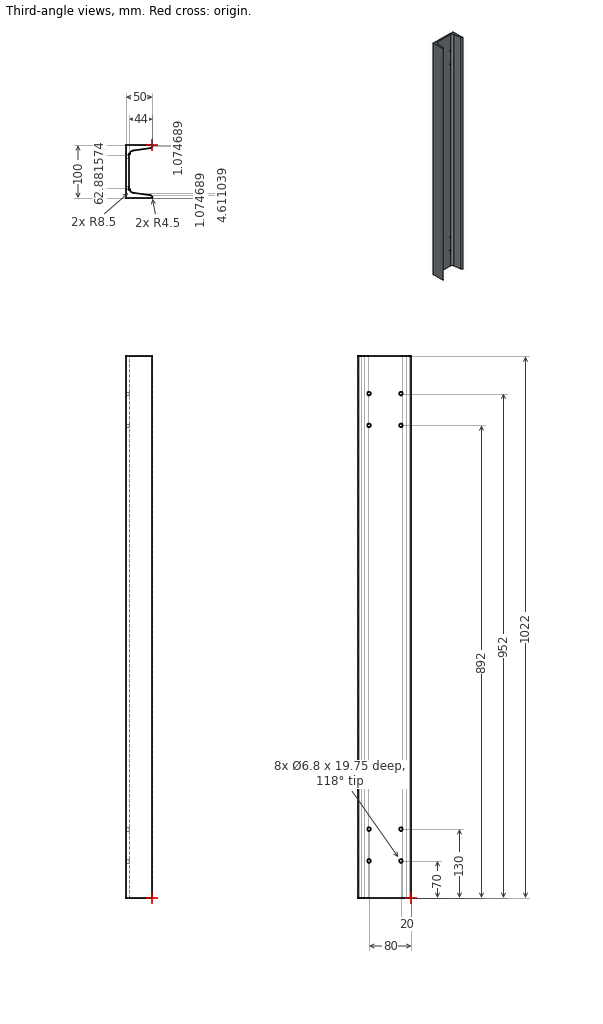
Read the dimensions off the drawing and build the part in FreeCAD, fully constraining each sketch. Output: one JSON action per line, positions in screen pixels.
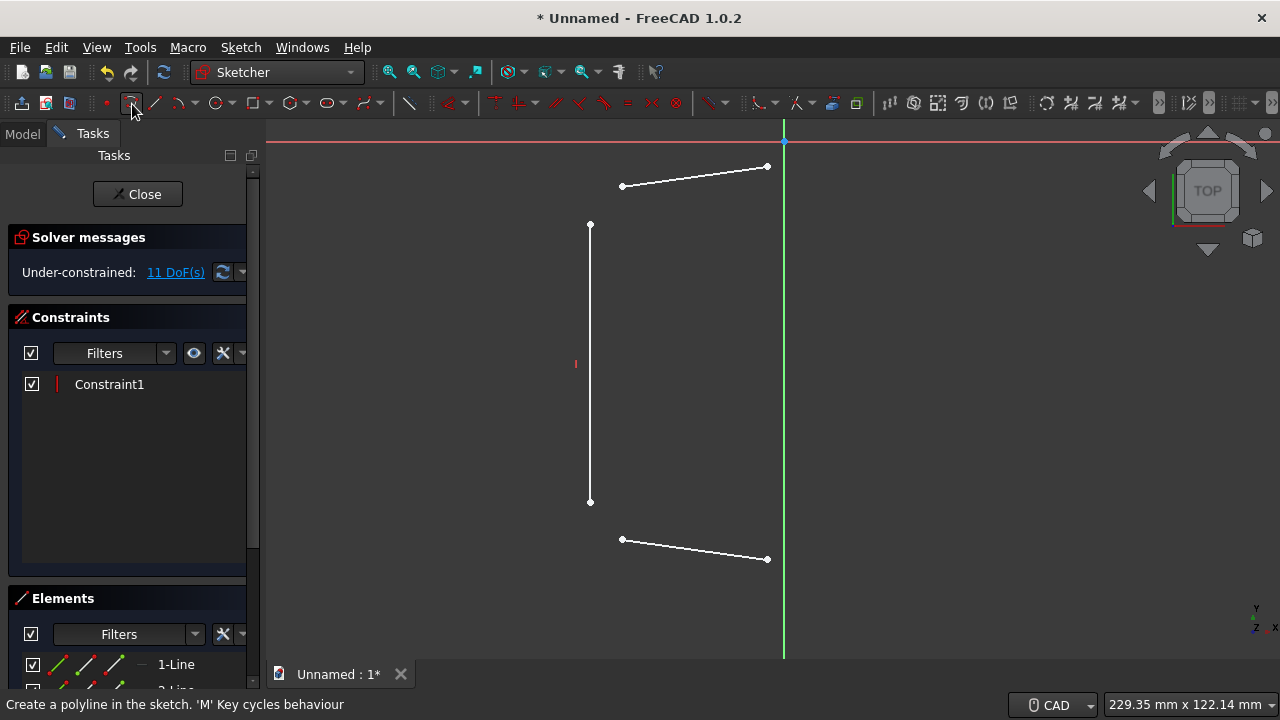
{"action": "scroll", "coordinate": [844, 508], "scroll_direction": "down", "scroll_amount": 1}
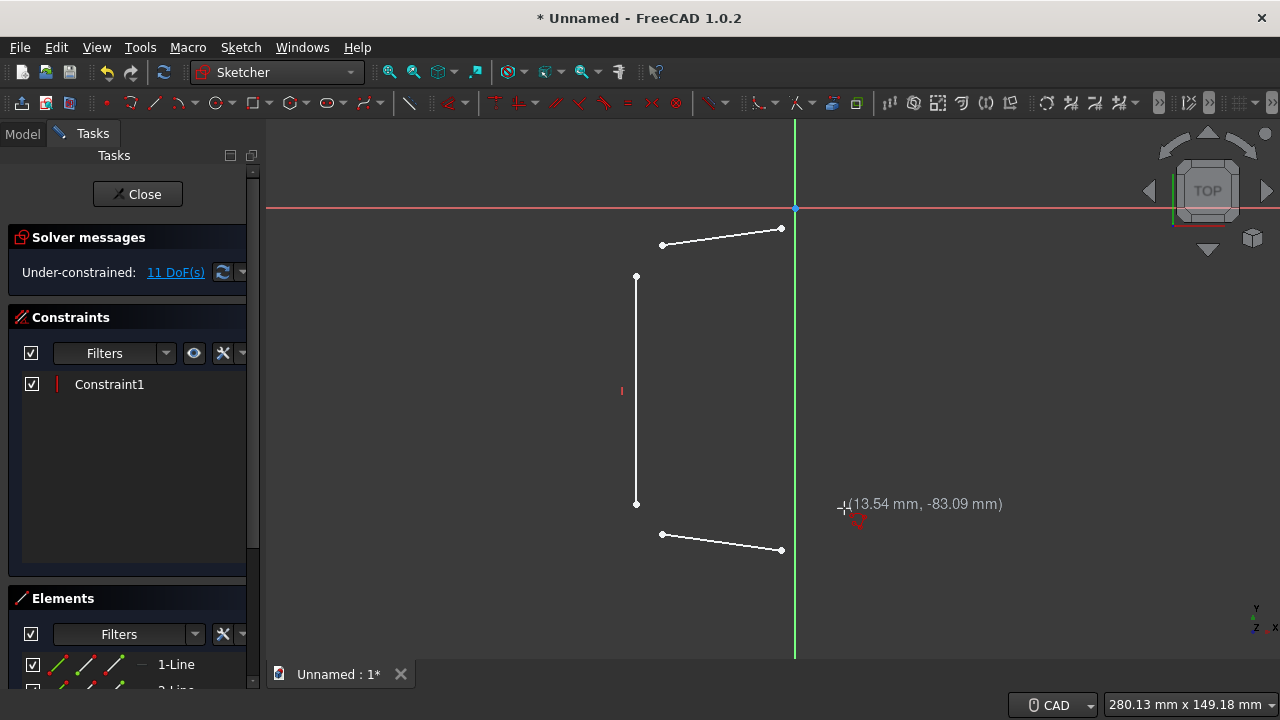
{"action": "scroll", "coordinate": [795, 212], "scroll_direction": "up", "scroll_amount": 8}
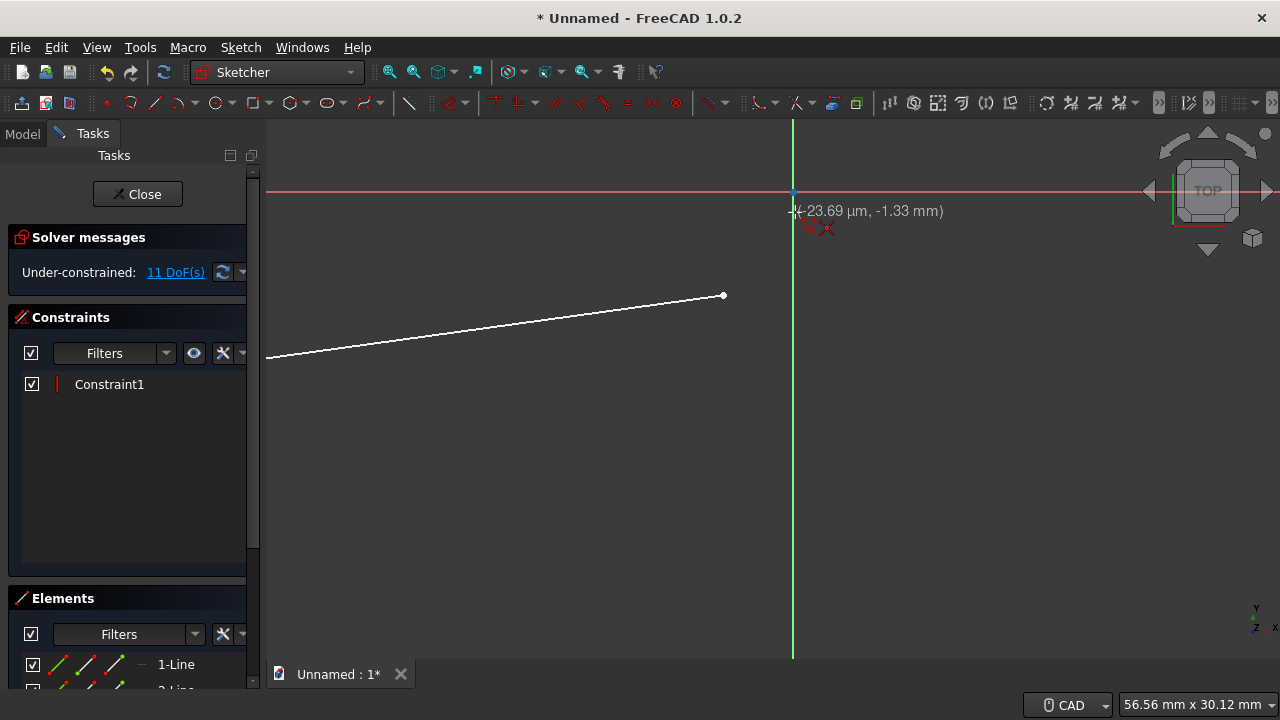
{"action": "left_click", "coordinate": [793, 212]}
{"action": "left_click", "coordinate": [793, 192]}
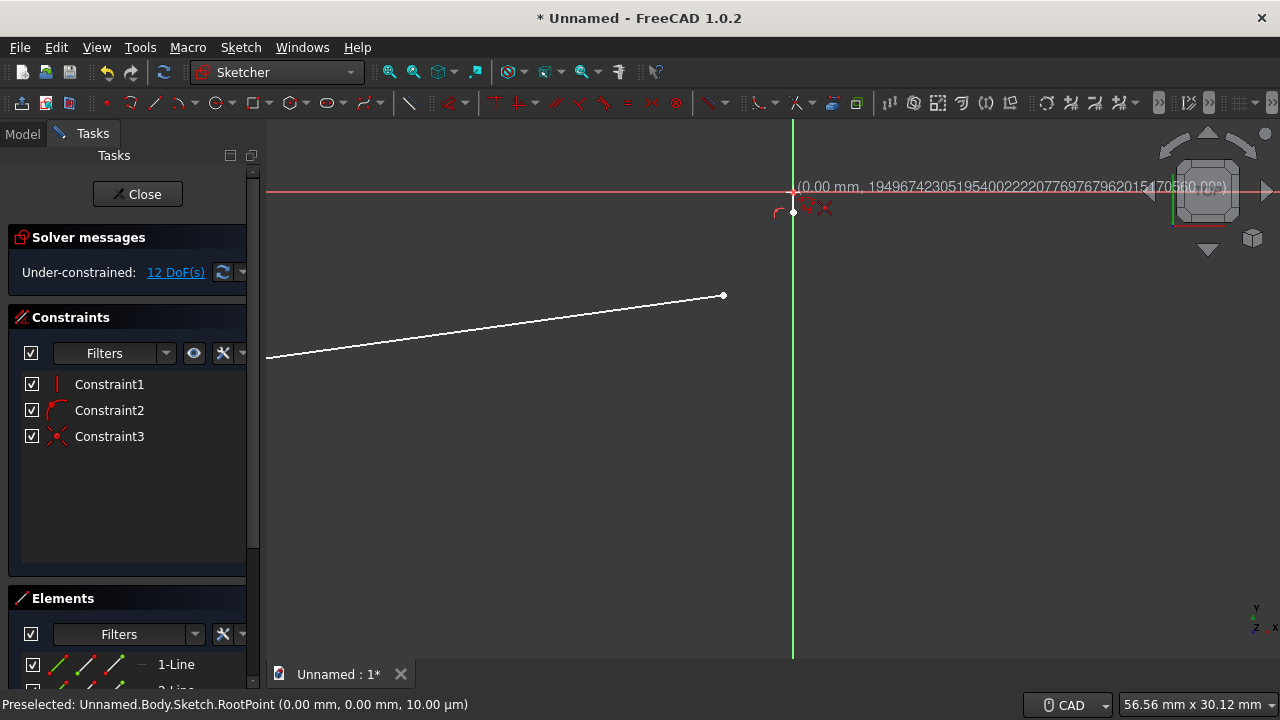
{"action": "scroll", "coordinate": [795, 212], "scroll_direction": "down", "scroll_amount": 8}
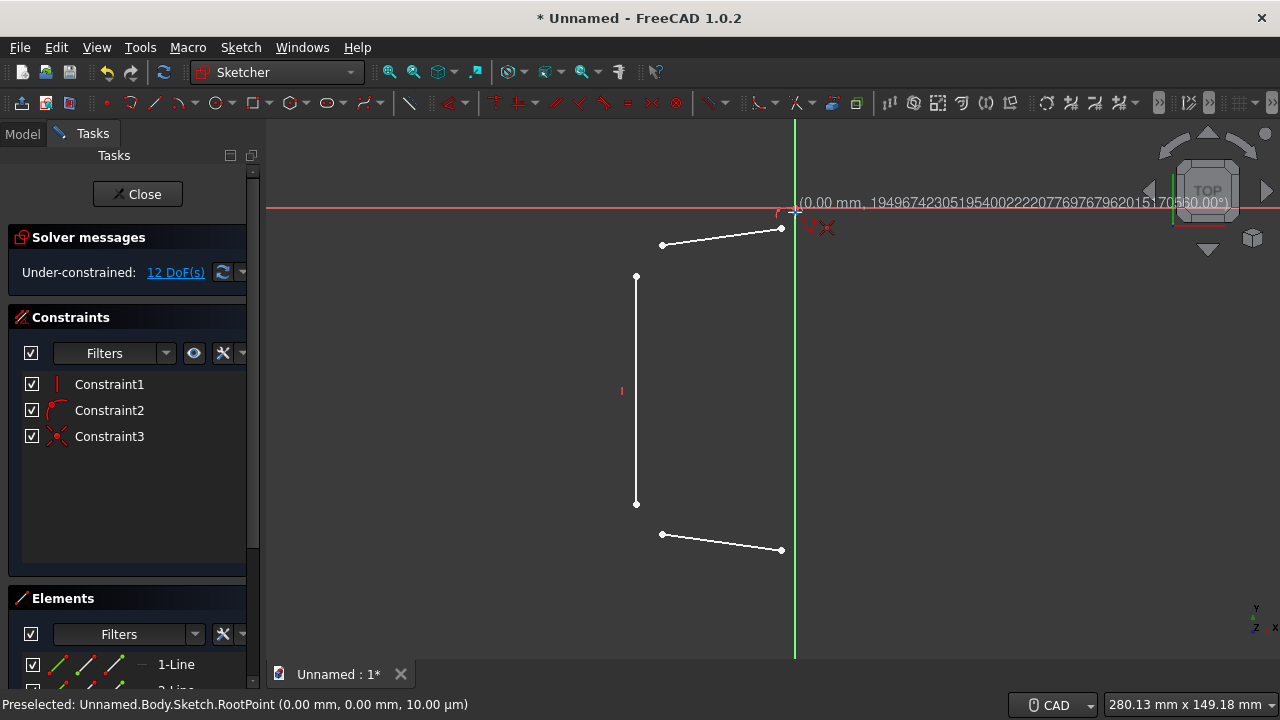
{"action": "left_click", "coordinate": [614, 217]}
{"action": "left_click", "coordinate": [614, 570]}
{"action": "left_click", "coordinate": [795, 570]}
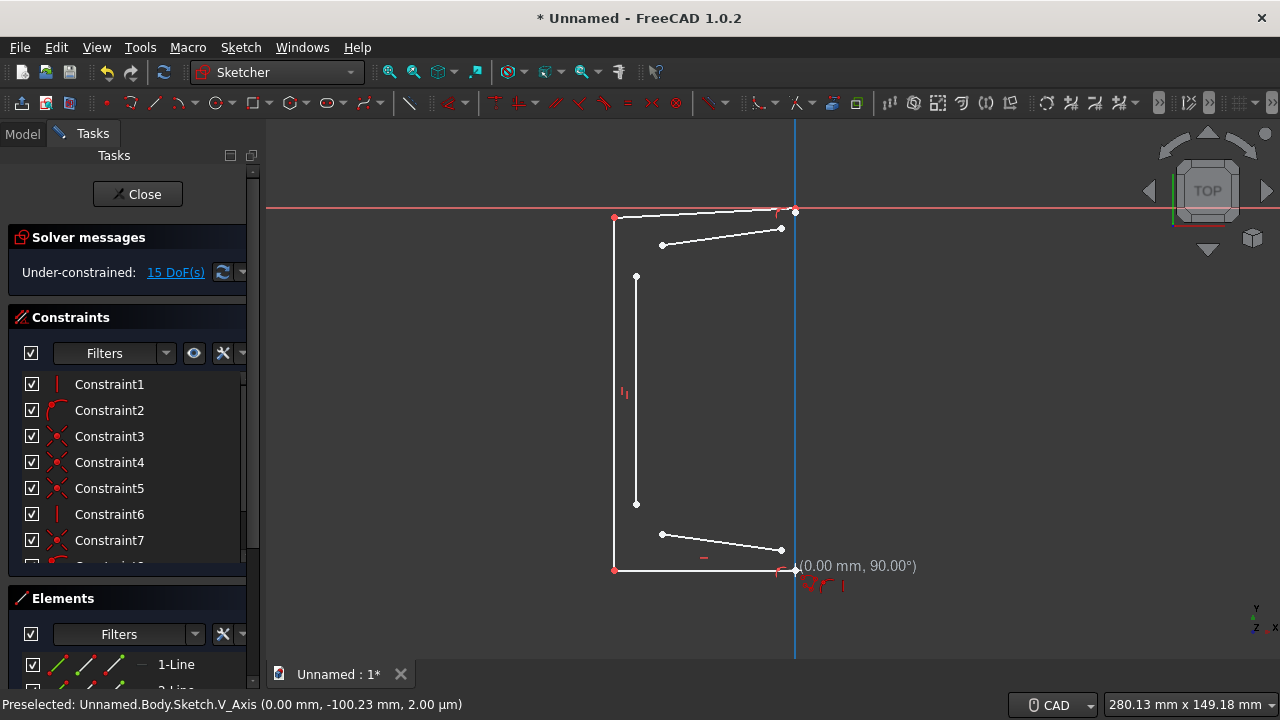
{"action": "scroll", "coordinate": [795, 566], "scroll_direction": "up", "scroll_amount": 8}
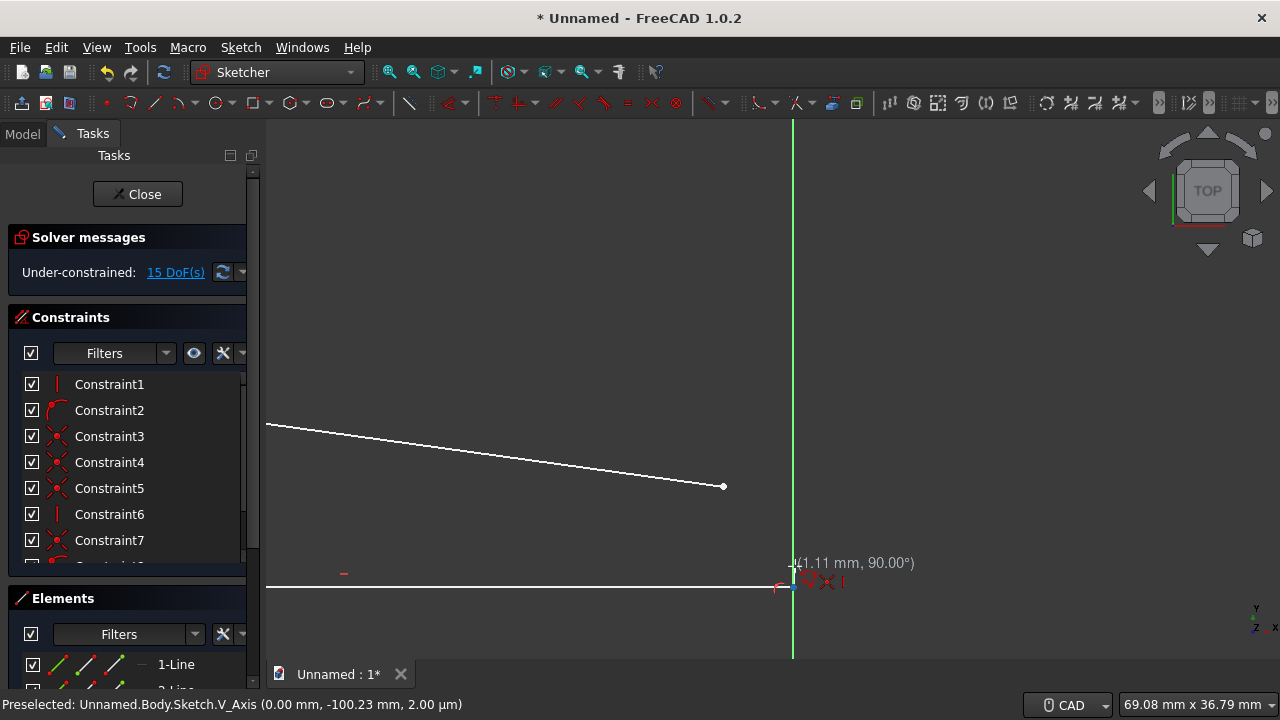
{"action": "left_click", "coordinate": [784, 564]}
{"action": "right_click", "coordinate": [784, 564]}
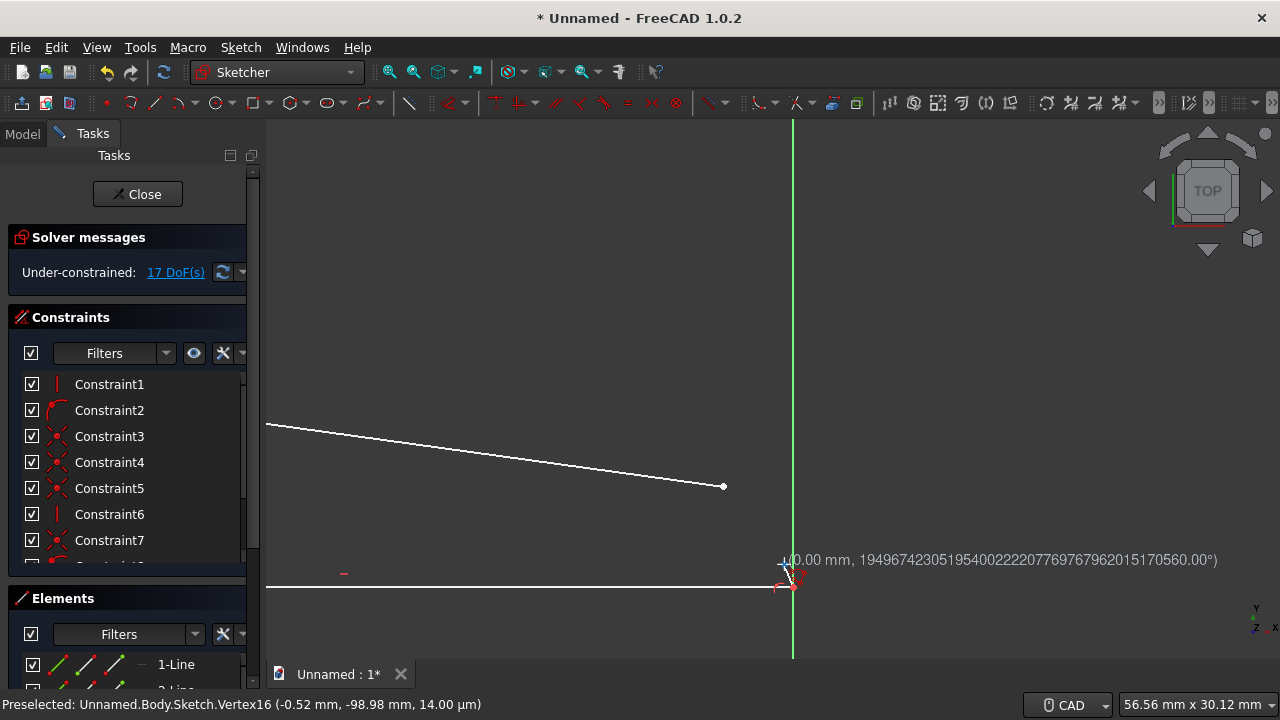
{"action": "key", "text": "g 3 a"}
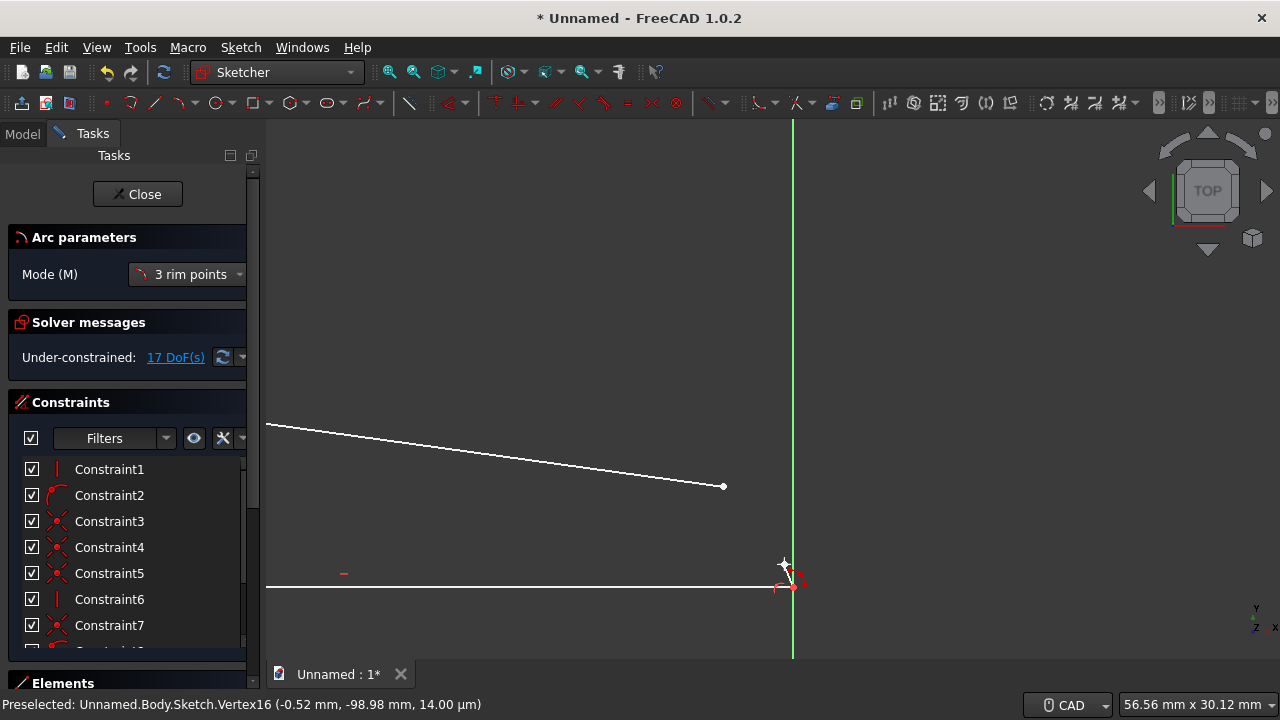
{"action": "scroll", "coordinate": [795, 567], "scroll_direction": "down", "scroll_amount": 8}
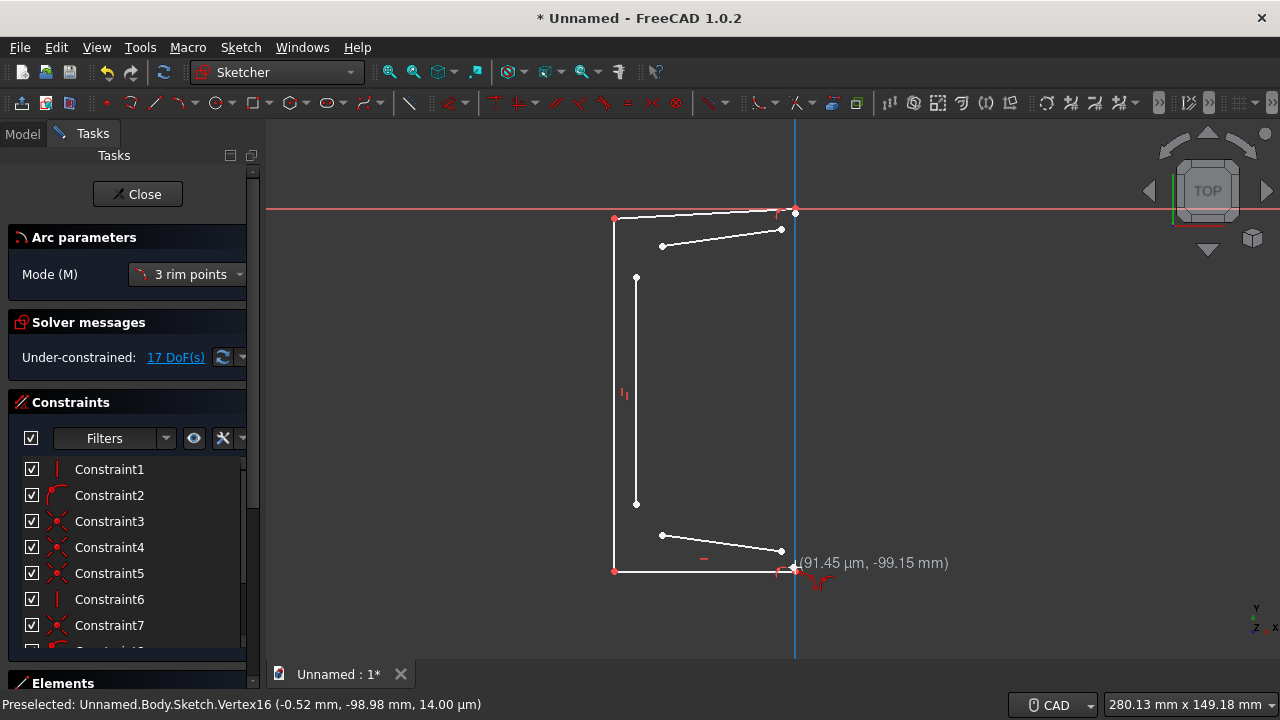
{"action": "left_click", "coordinate": [662, 535]}
{"action": "left_click", "coordinate": [636, 505]}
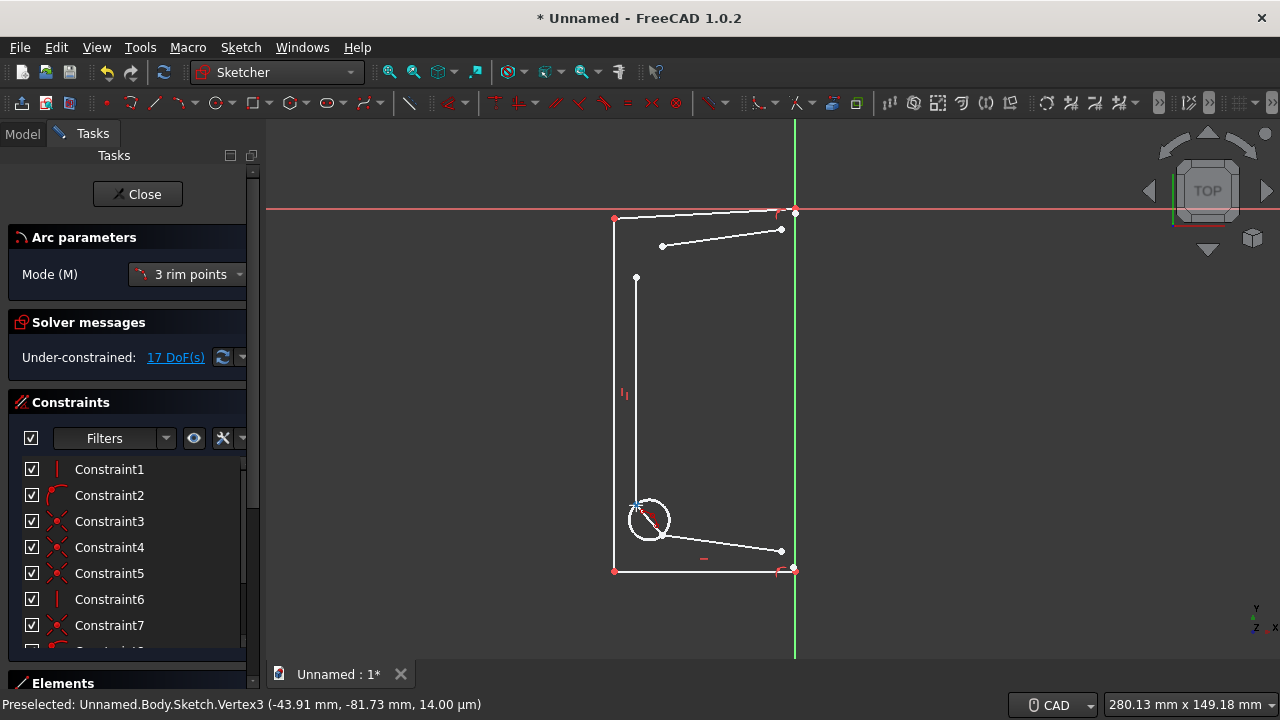
{"action": "scroll", "coordinate": [643, 524], "scroll_direction": "up", "scroll_amount": 4}